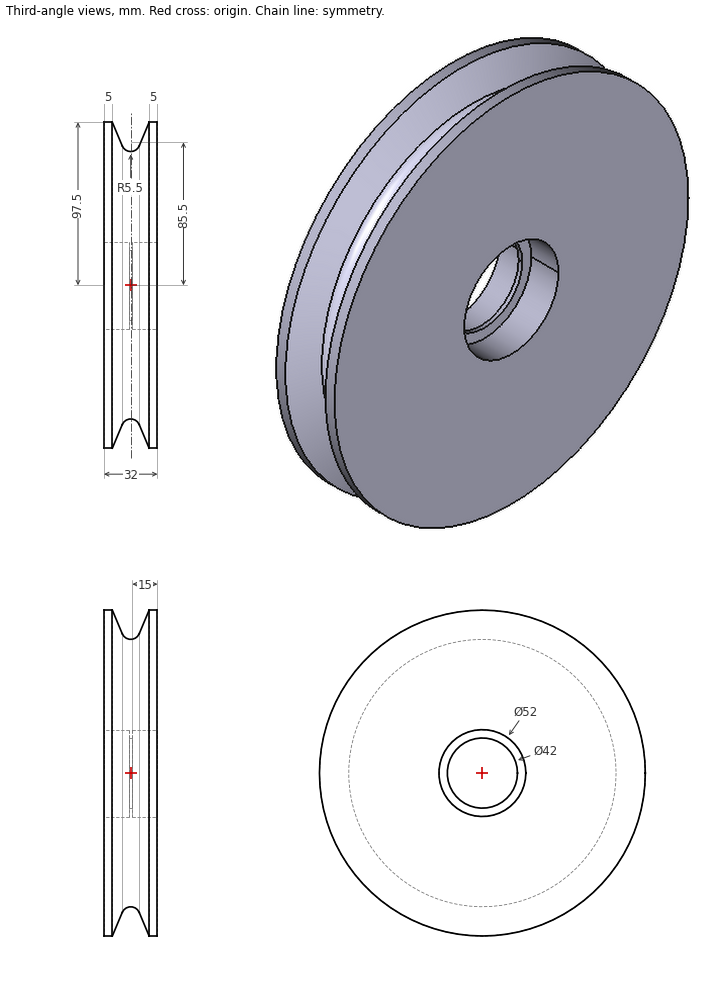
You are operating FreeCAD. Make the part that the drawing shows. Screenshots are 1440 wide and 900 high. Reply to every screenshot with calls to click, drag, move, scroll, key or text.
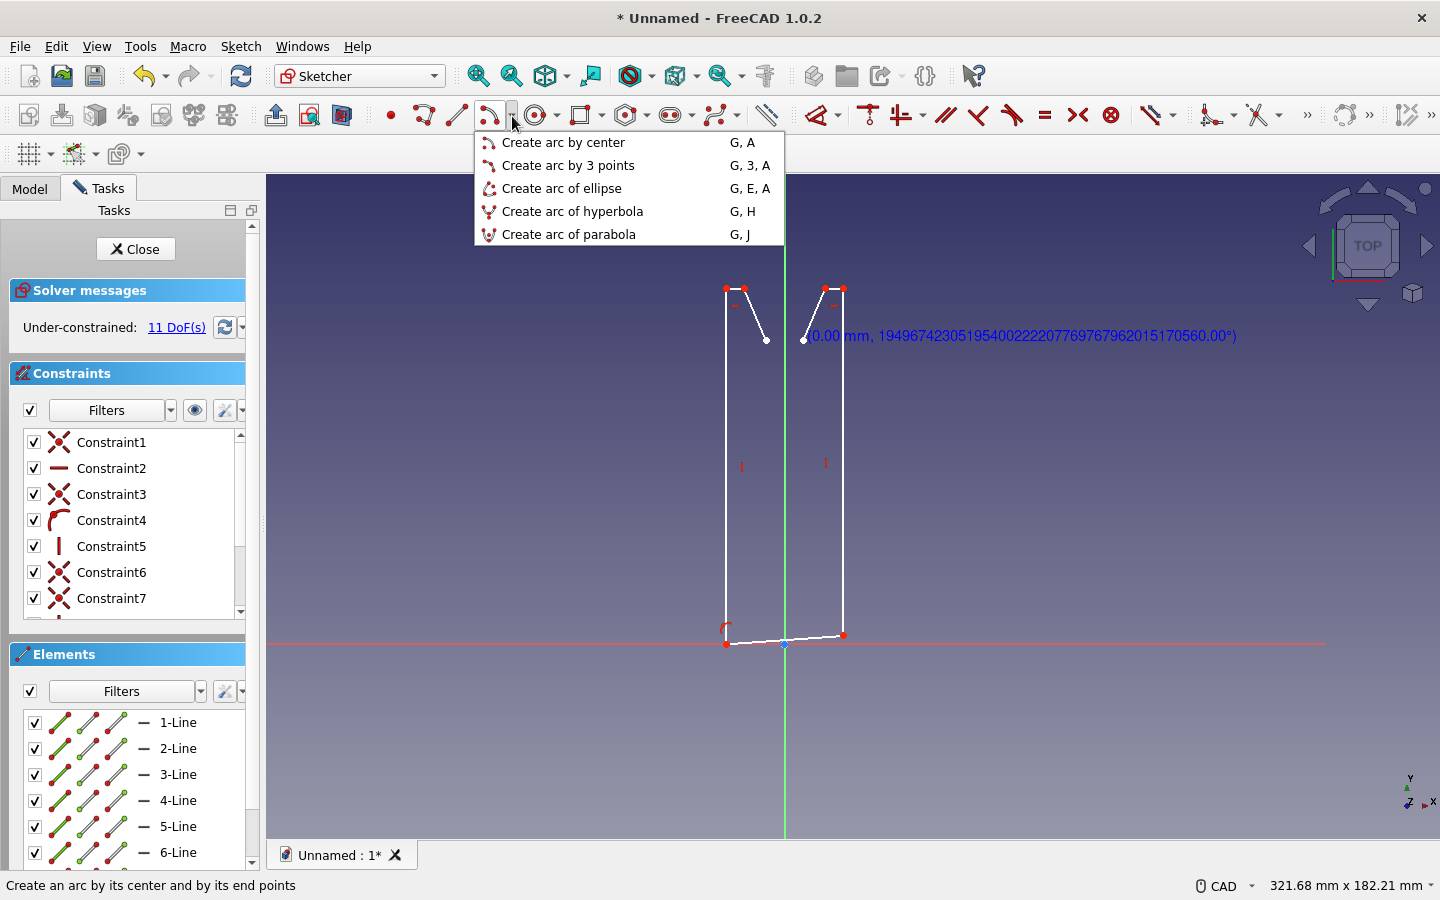
click(630, 166)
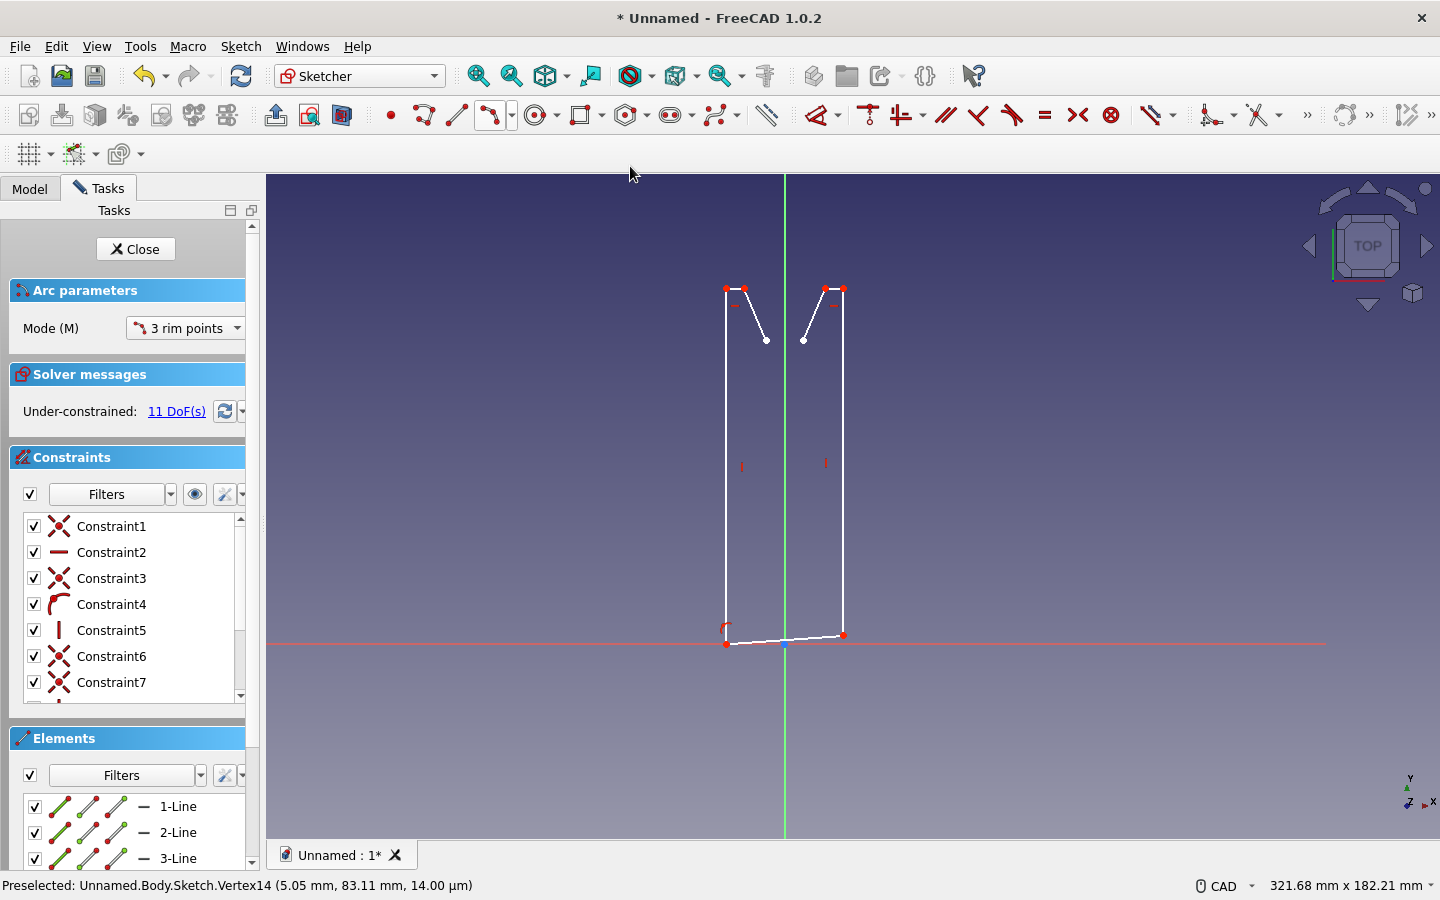
click(803, 341)
click(766, 341)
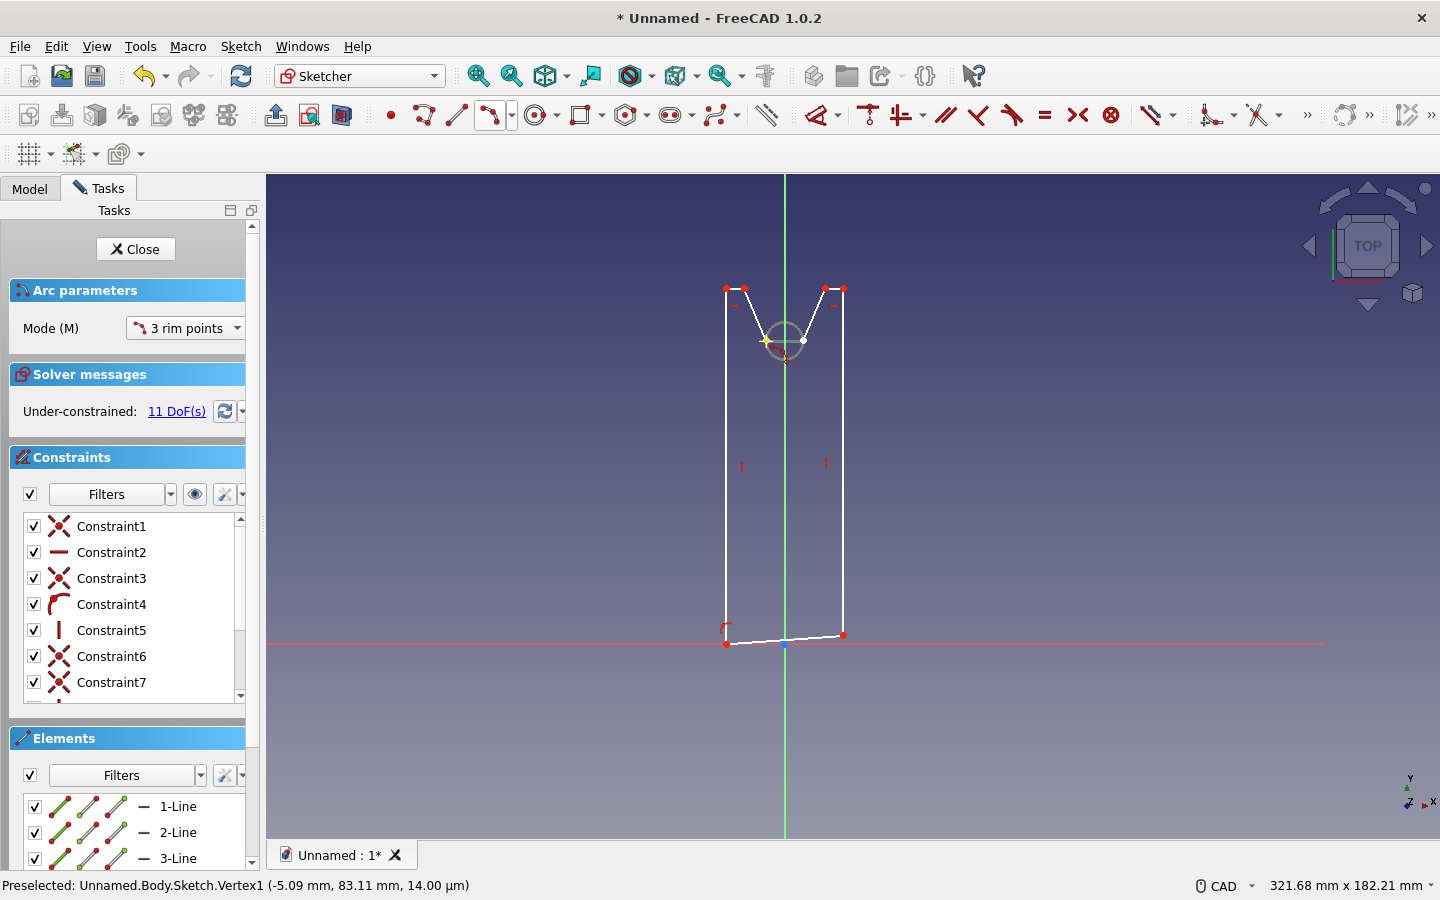
scroll(776, 350, up, 3)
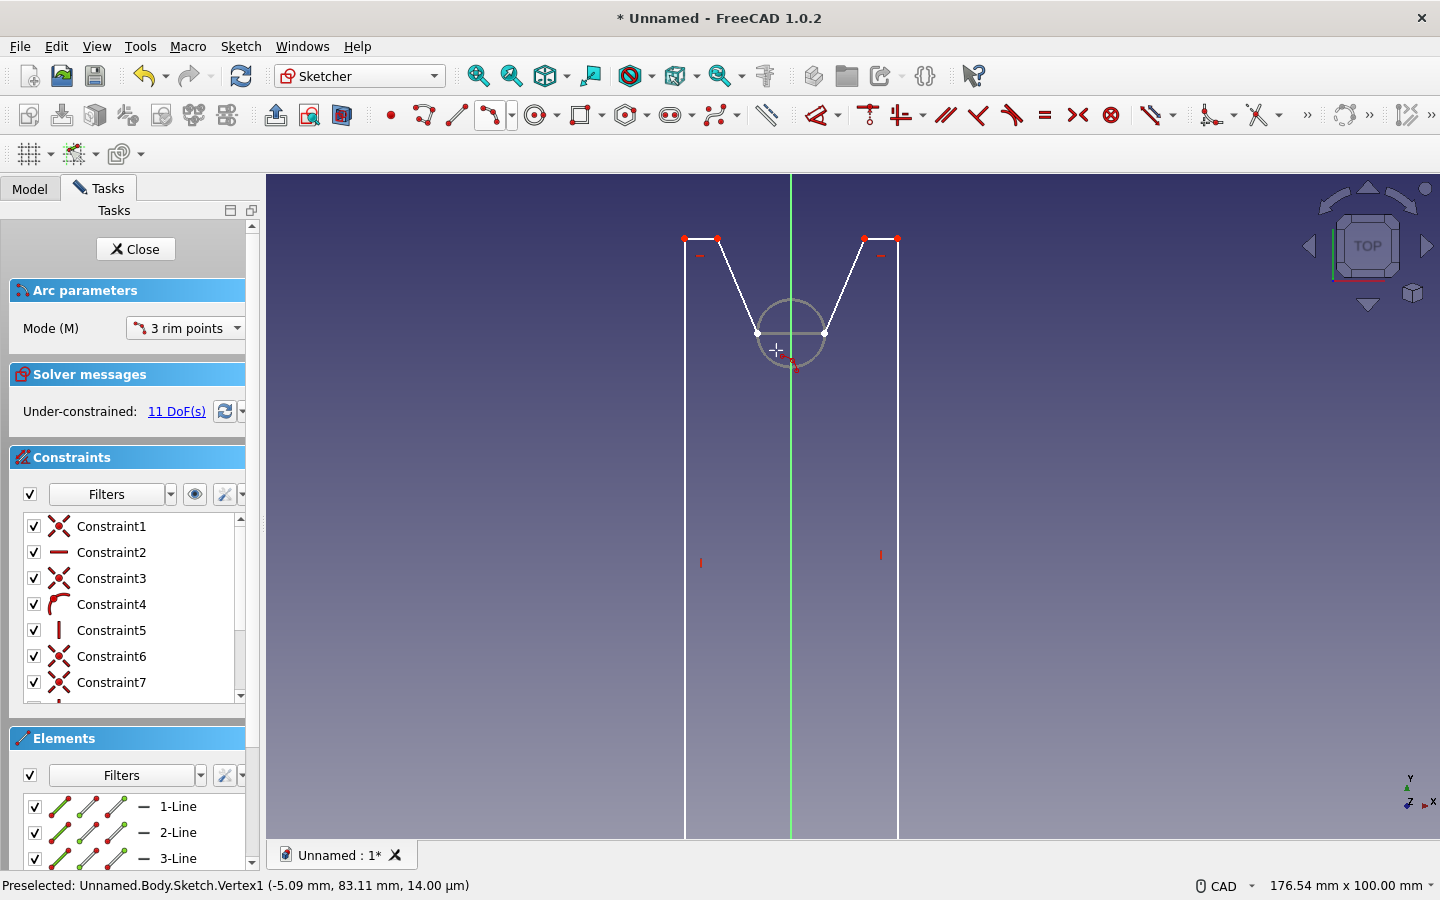
click(775, 350)
key(Escape)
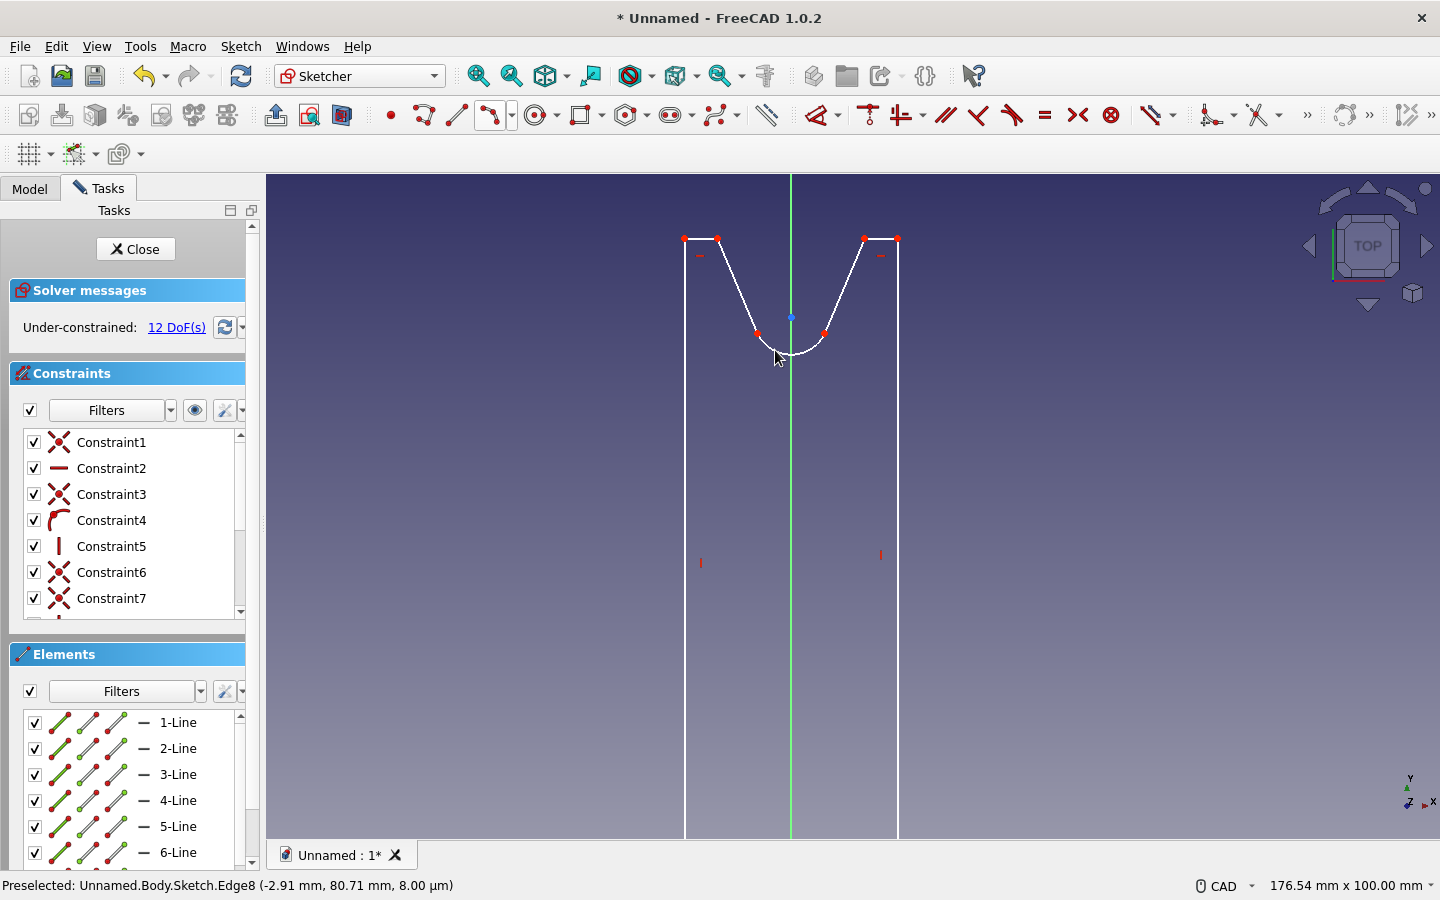
click(745, 305)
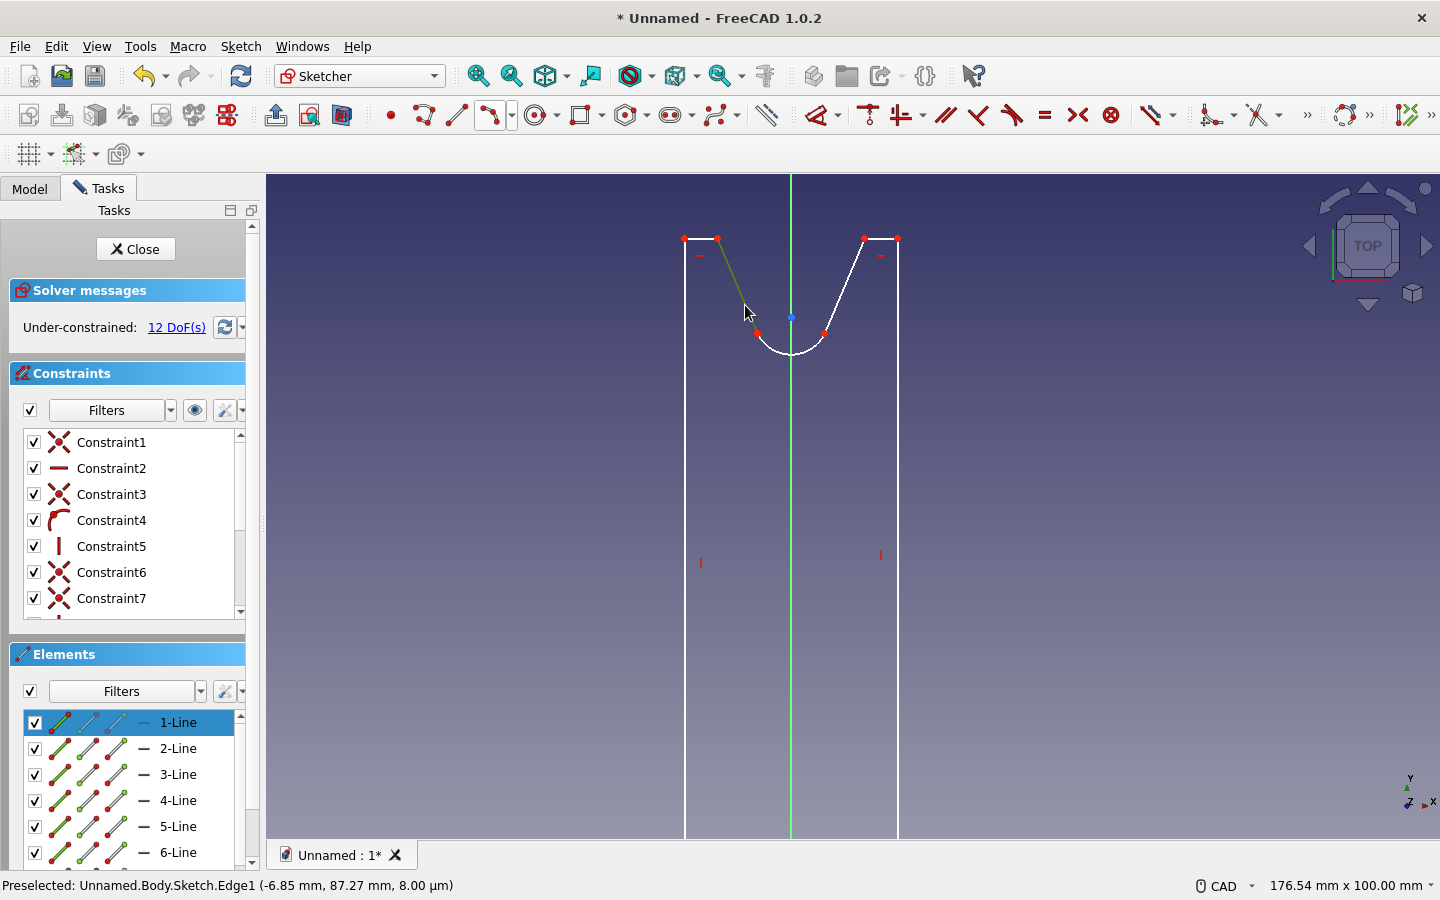
click(775, 351)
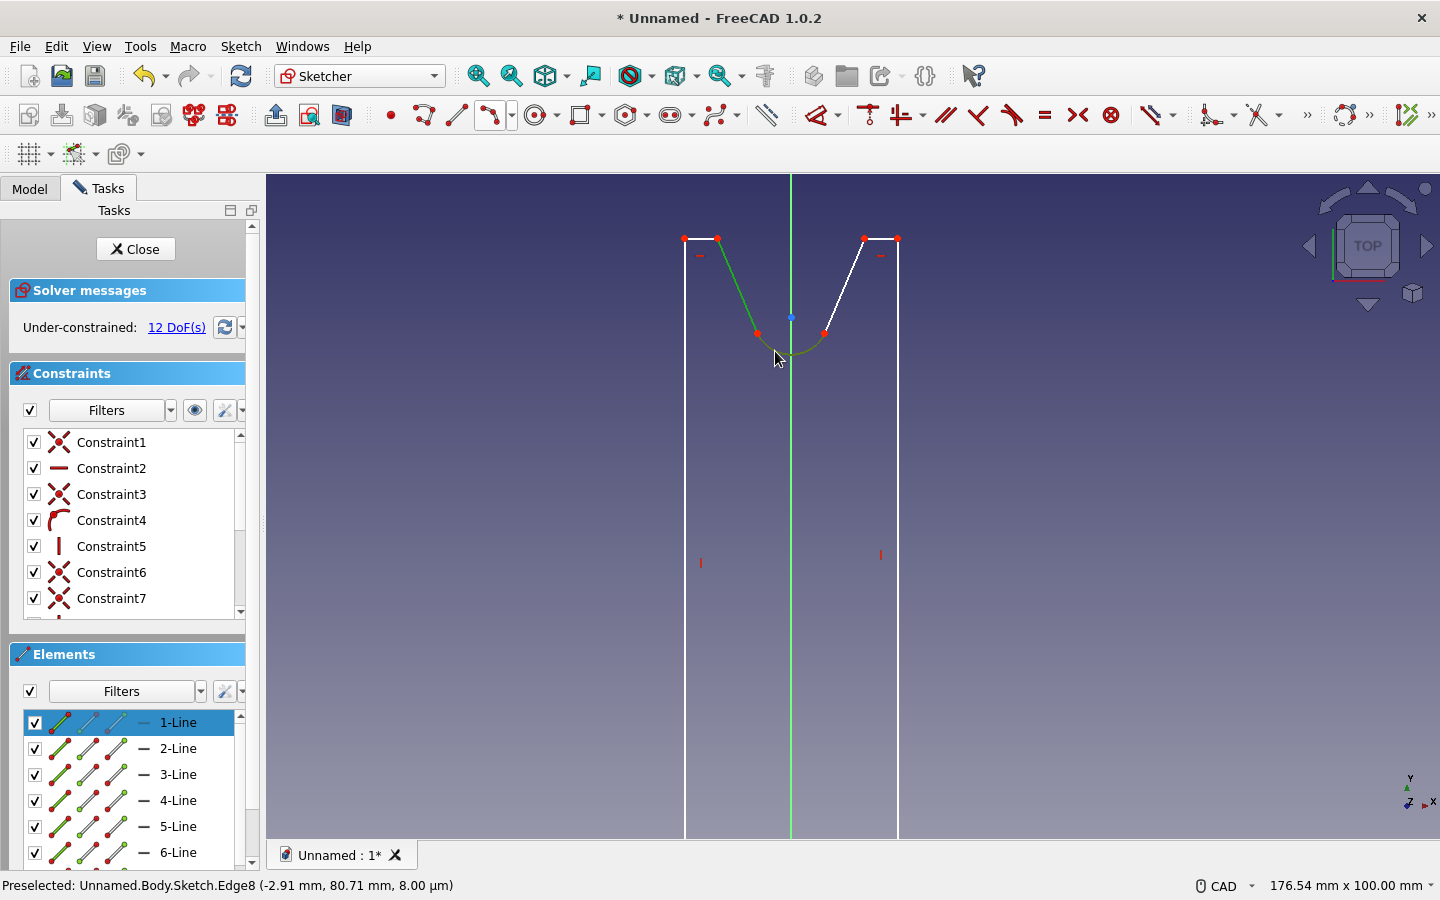
click(1012, 116)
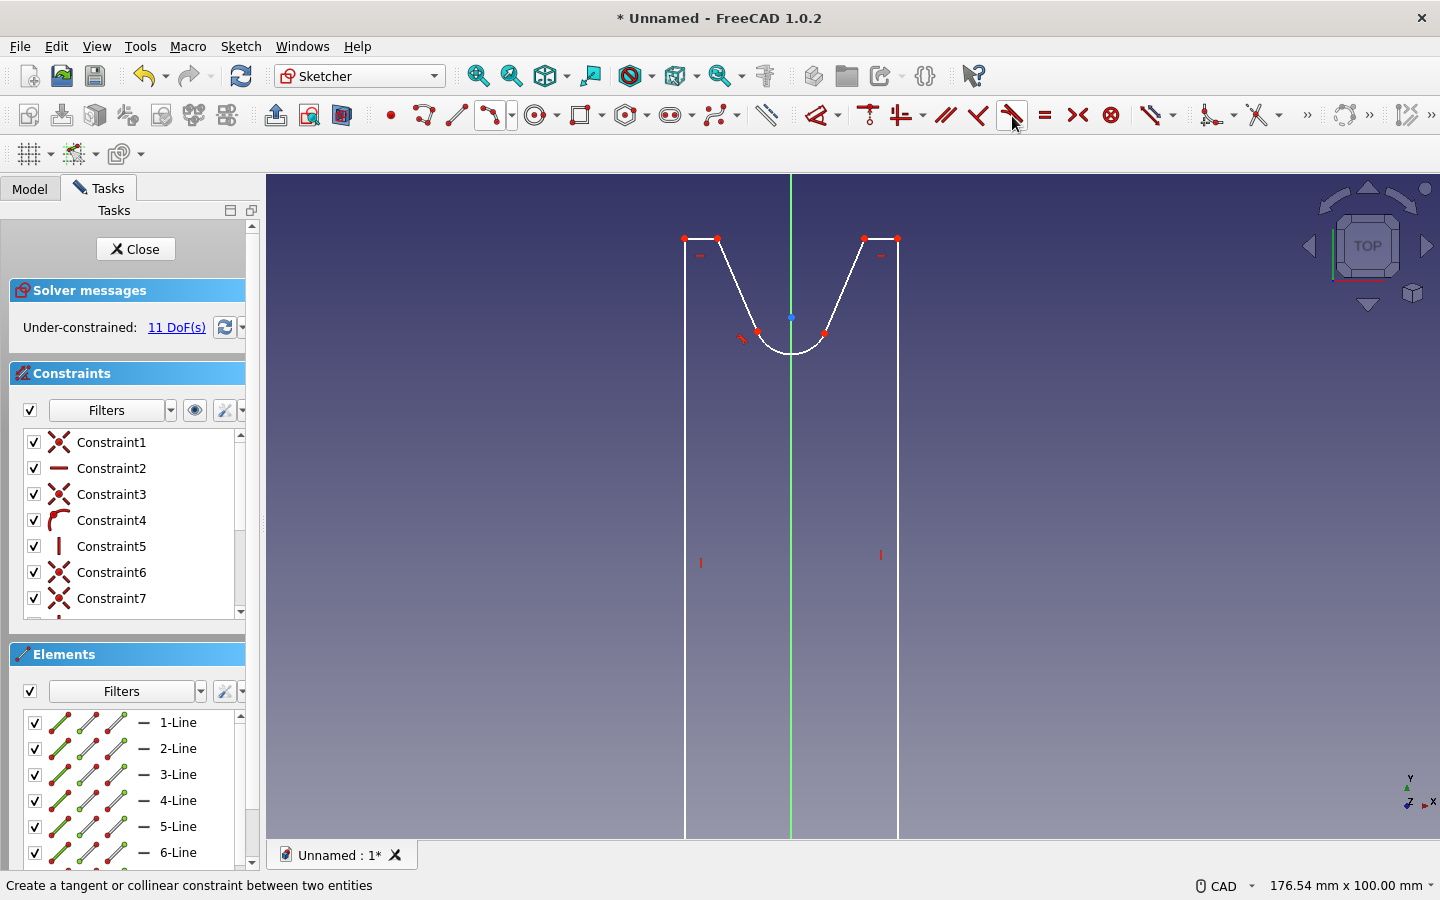
click(853, 267)